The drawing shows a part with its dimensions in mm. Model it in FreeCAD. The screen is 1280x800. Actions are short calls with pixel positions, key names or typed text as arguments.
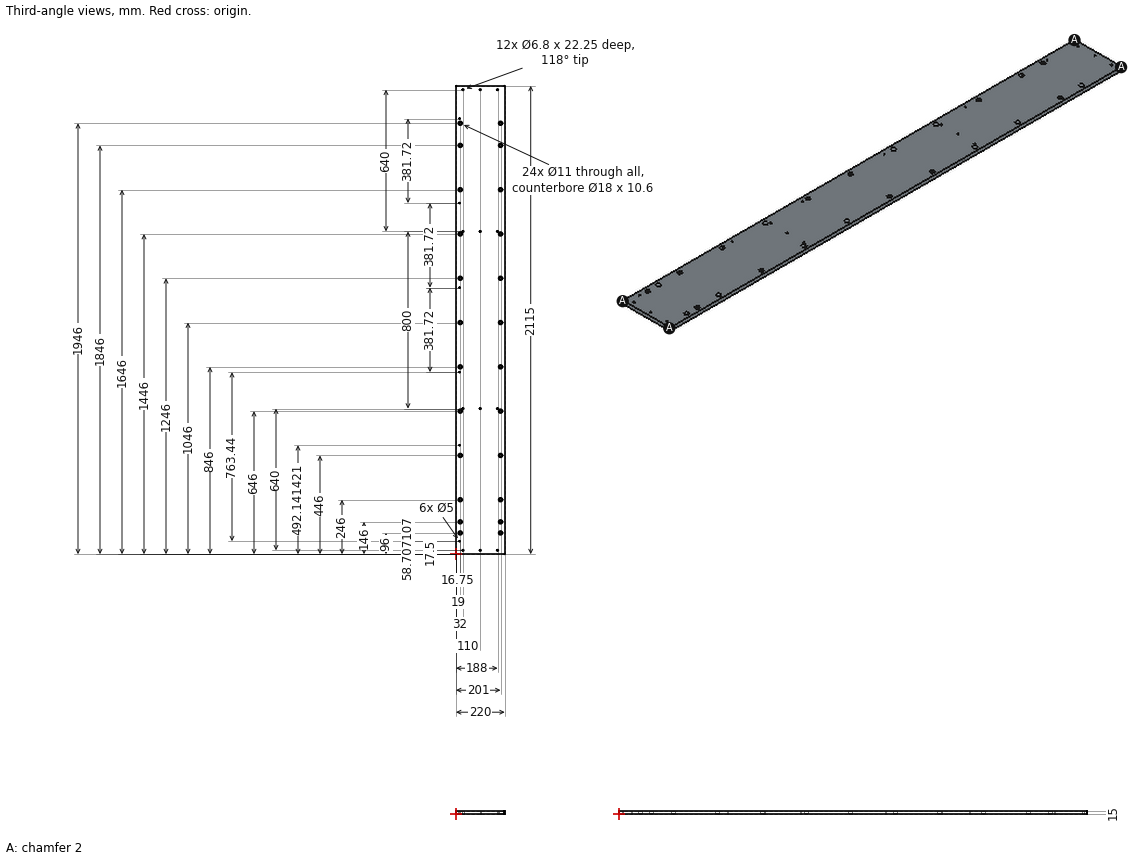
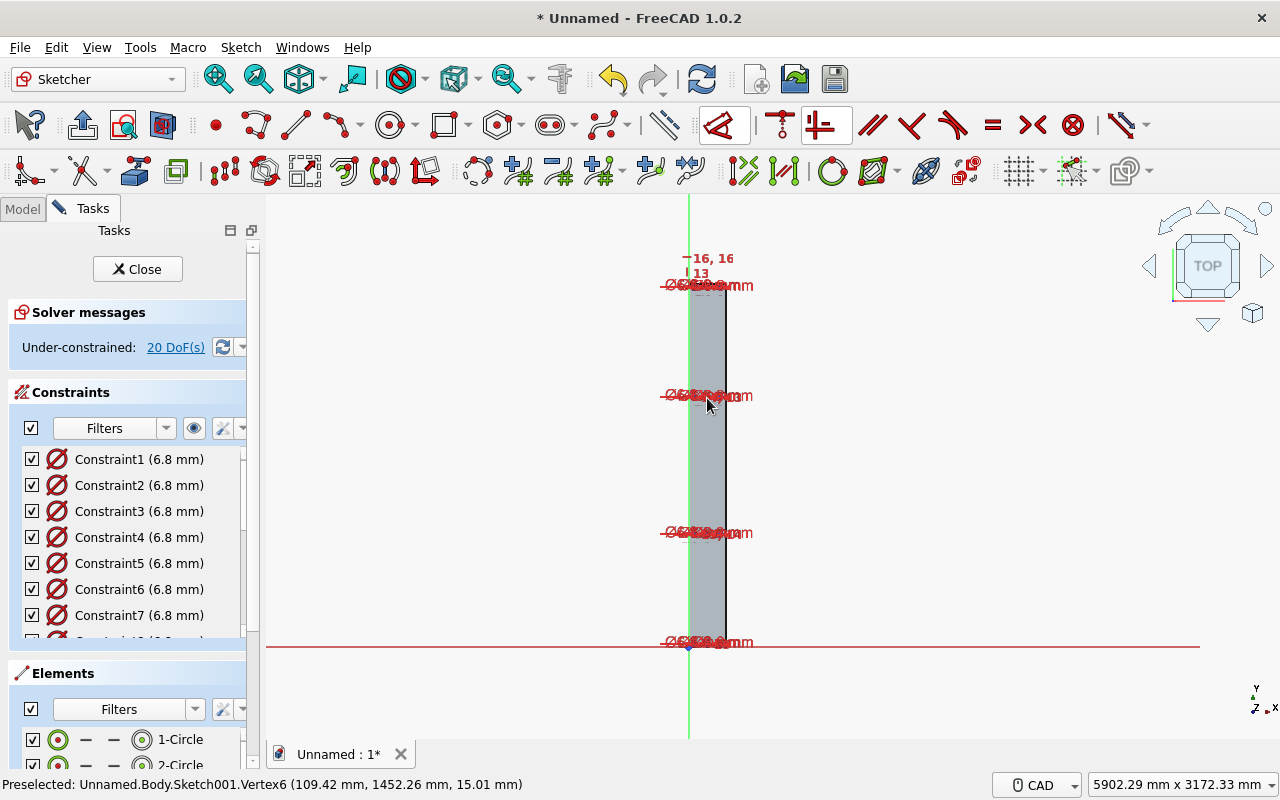
click(846, 126)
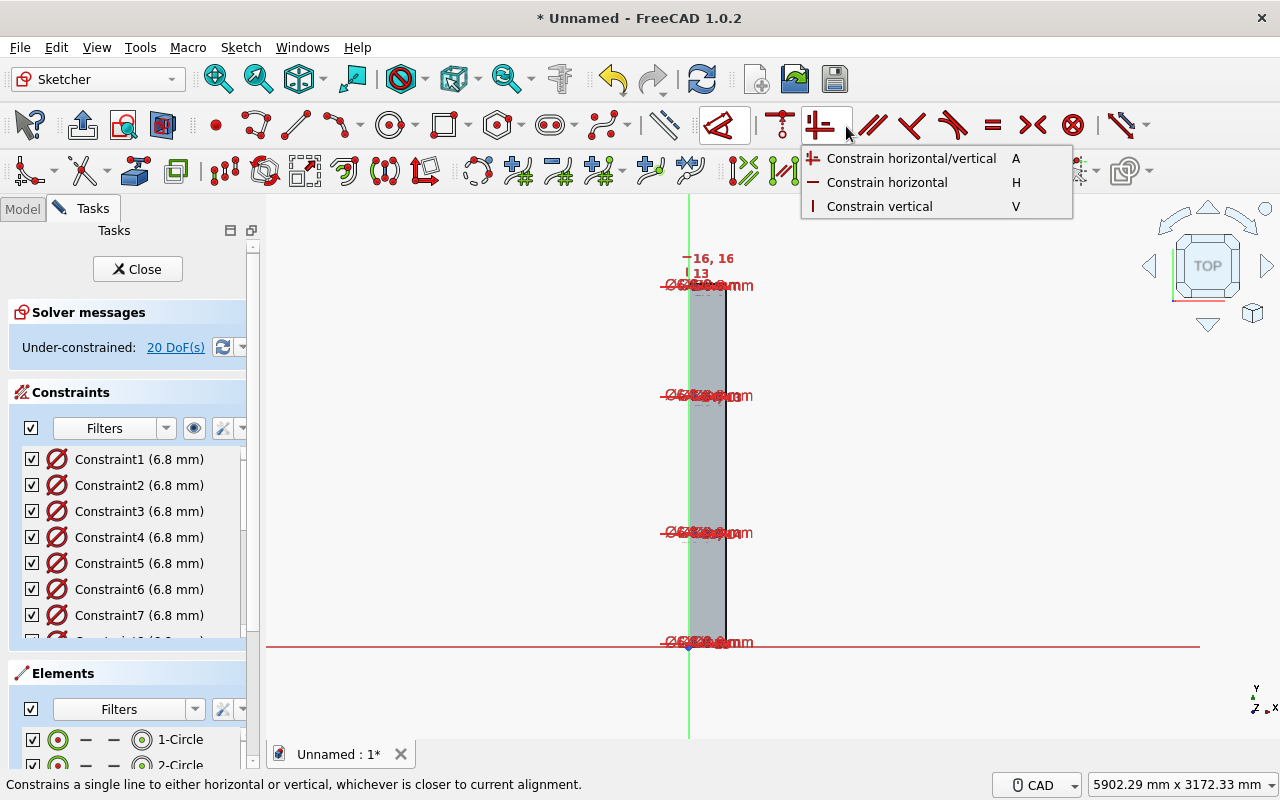
click(937, 206)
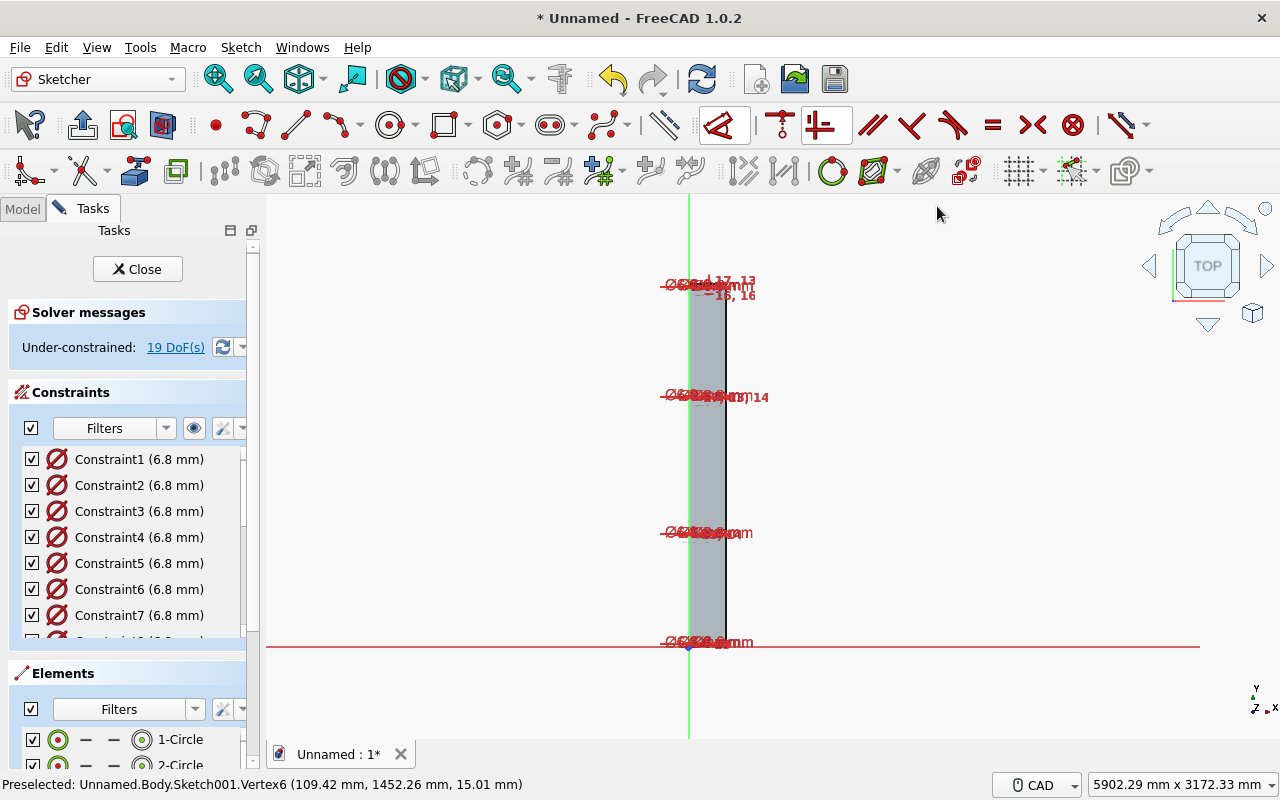
scroll(694, 397, up, 4)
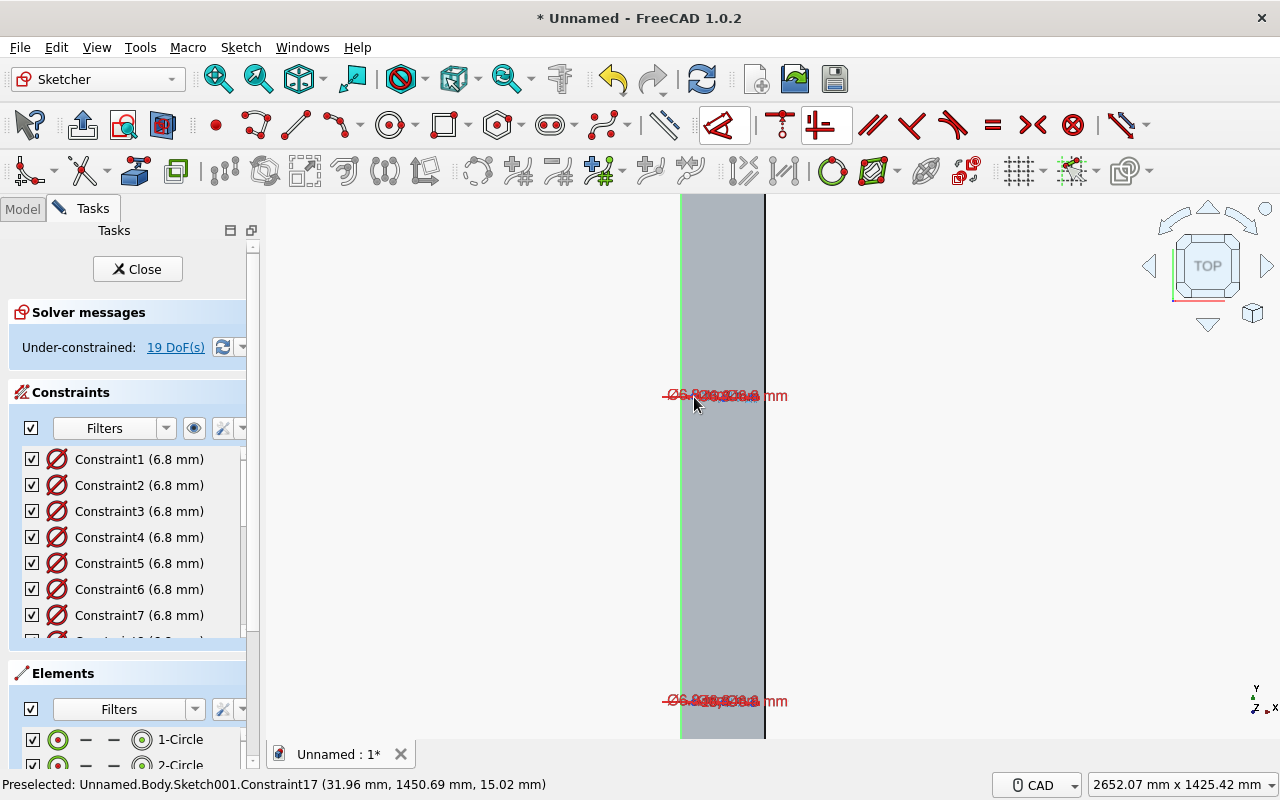
click(693, 397)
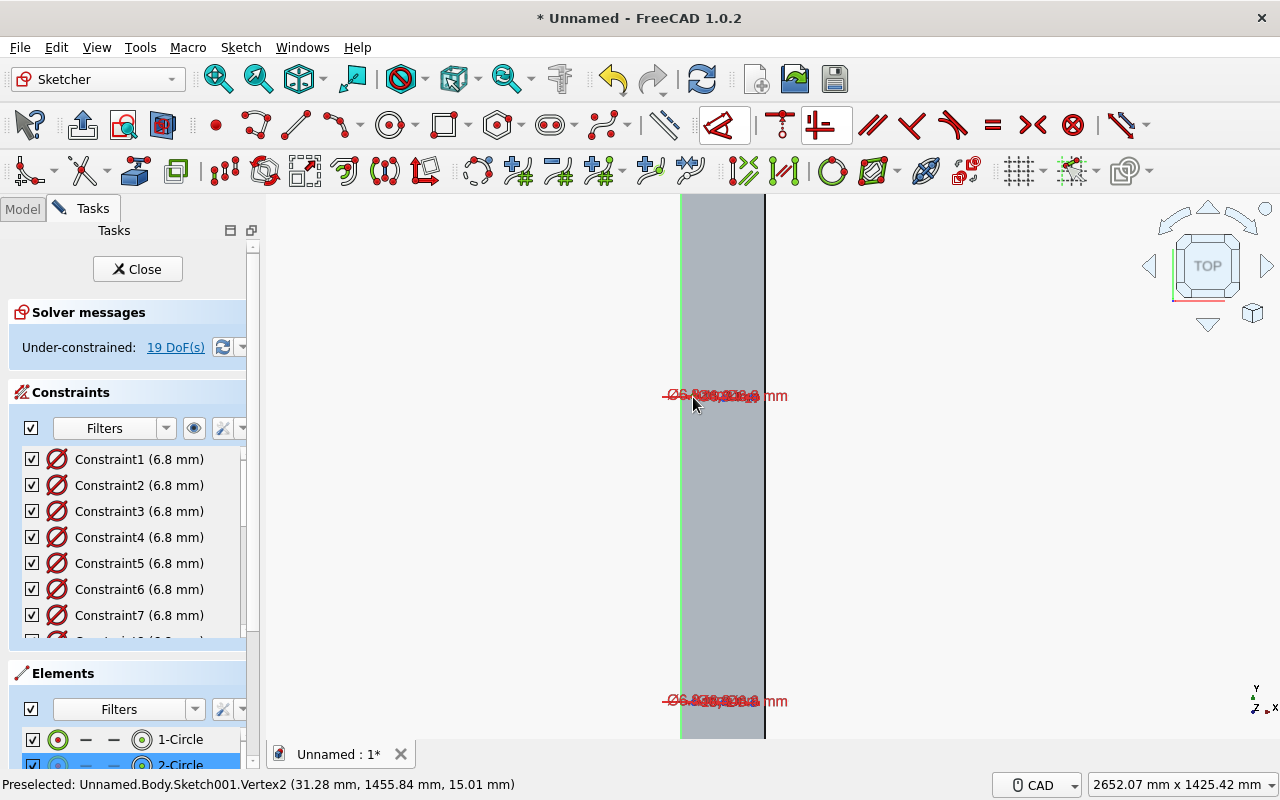
click(724, 398)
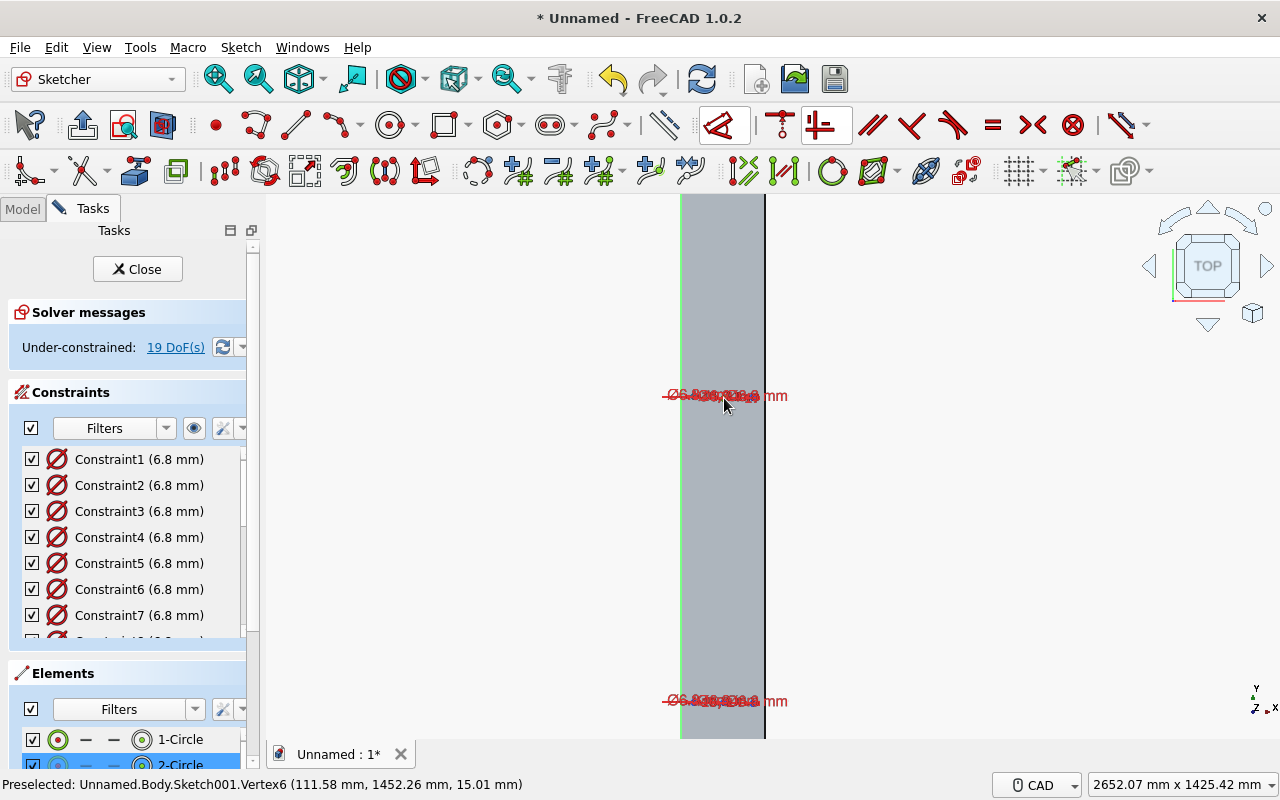
key(h)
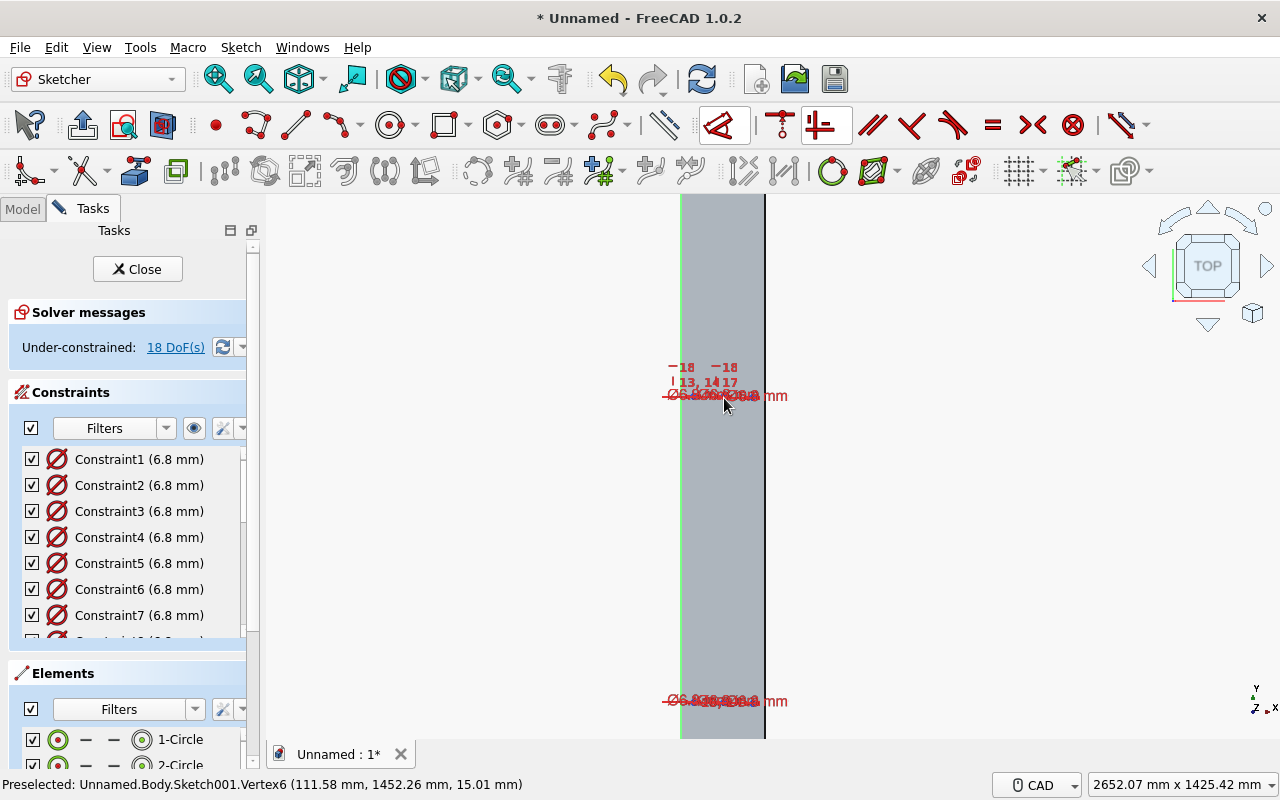
click(724, 397)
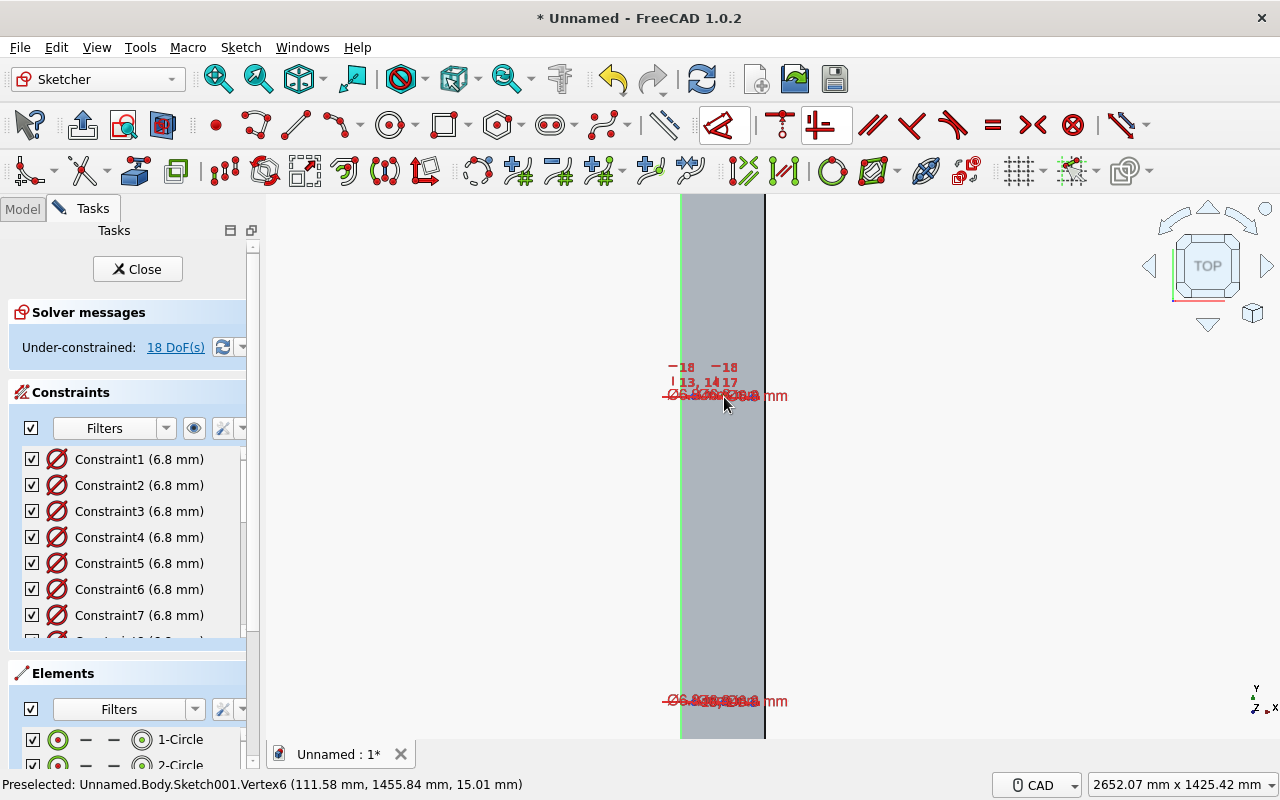
click(723, 703)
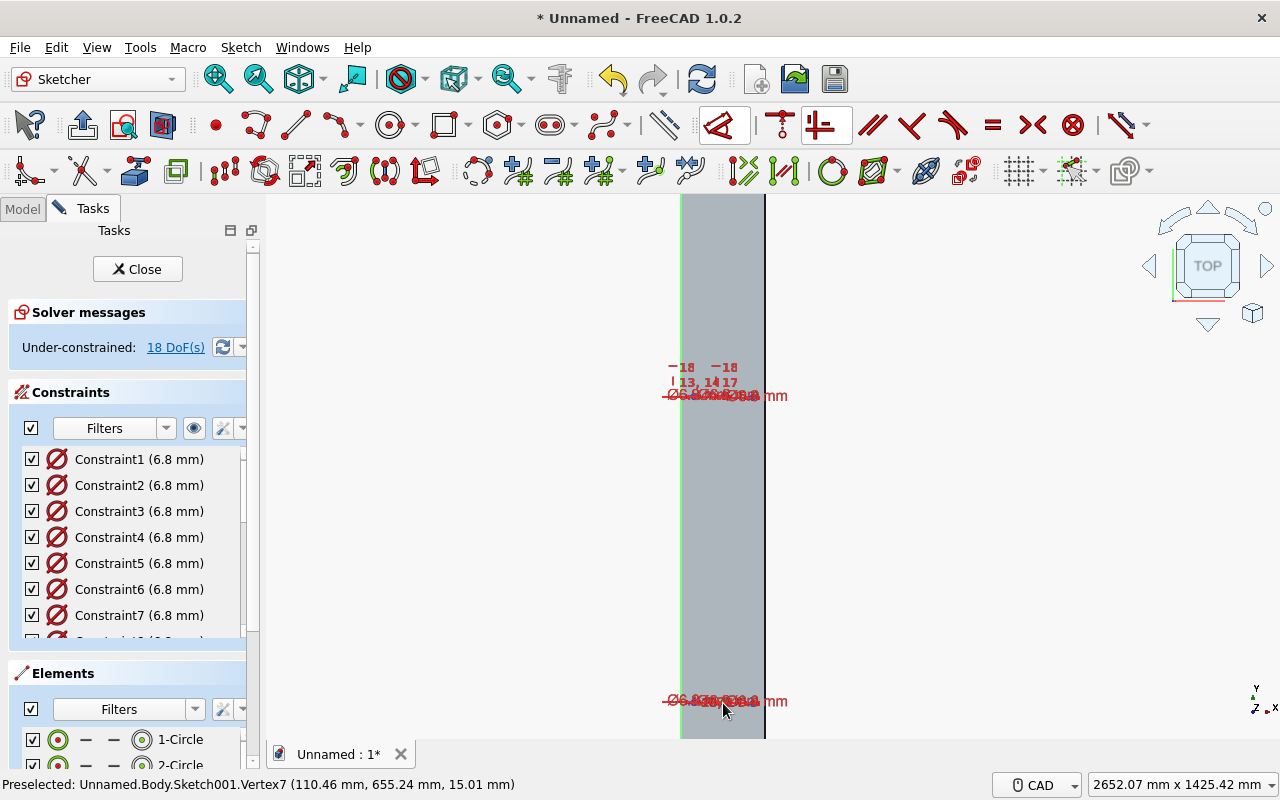
key(v)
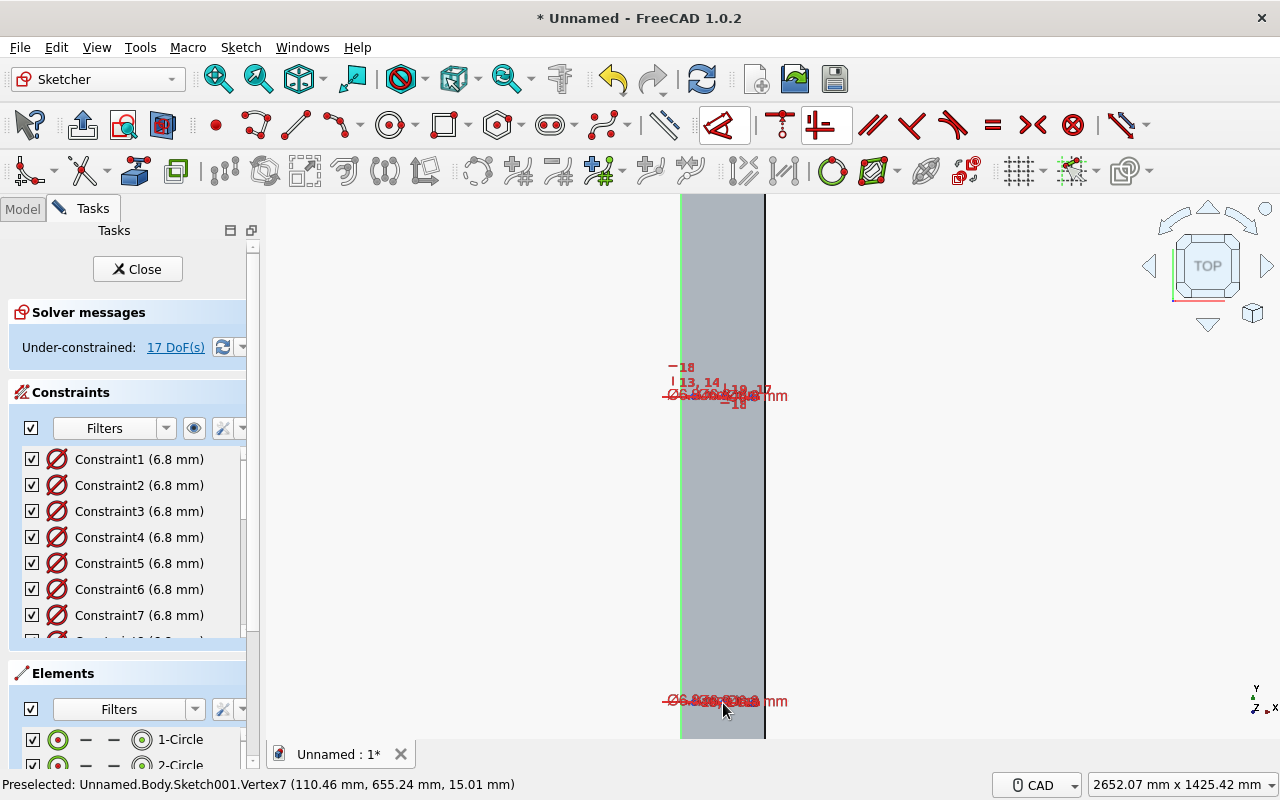
click(693, 702)